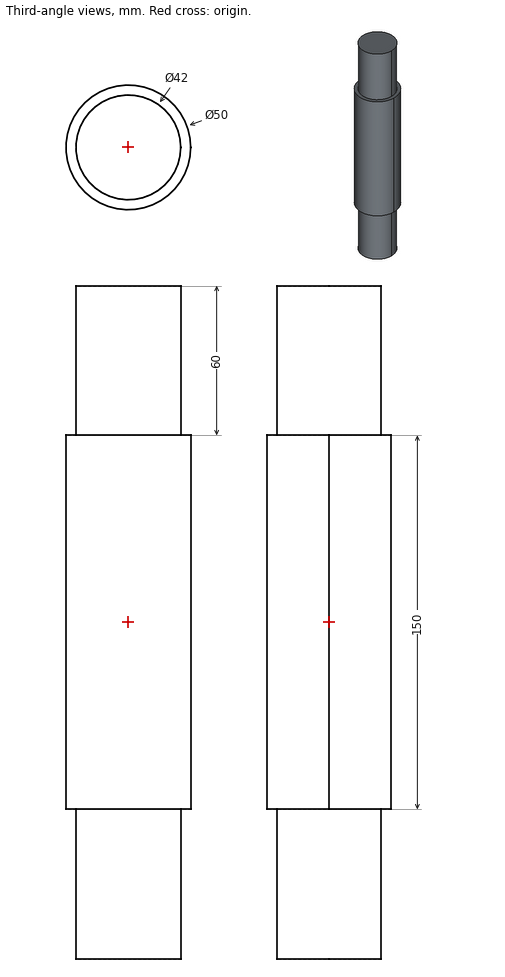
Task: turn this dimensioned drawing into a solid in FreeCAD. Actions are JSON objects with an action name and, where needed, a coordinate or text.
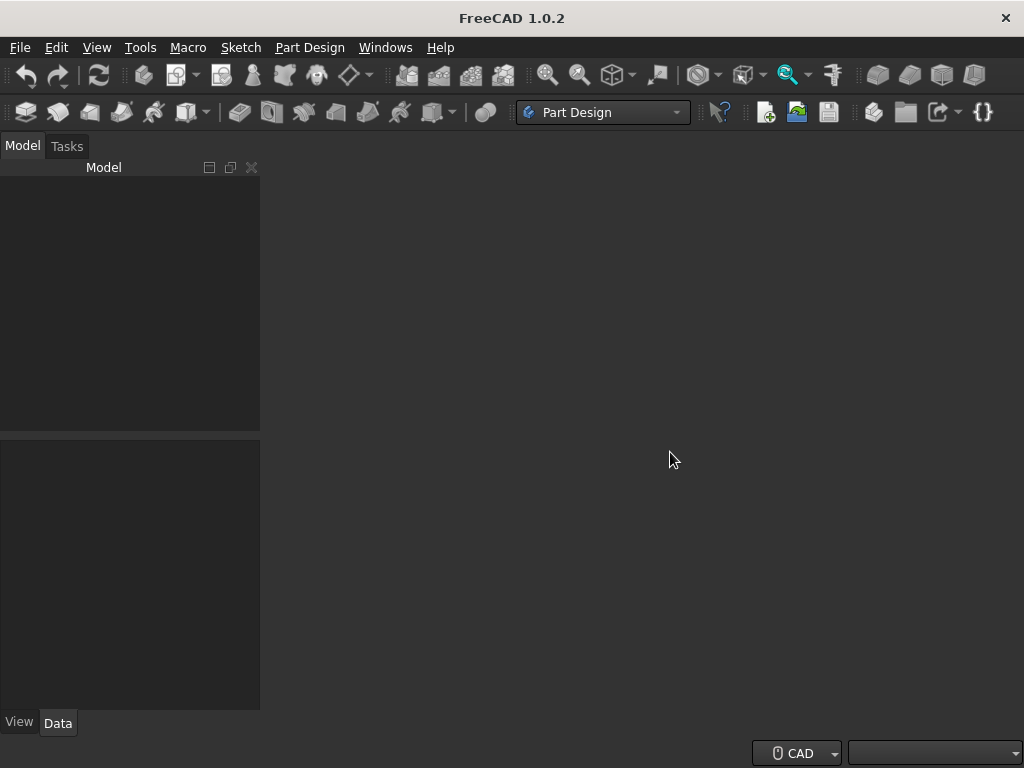
{"action": "left_click", "coordinate": [766, 112]}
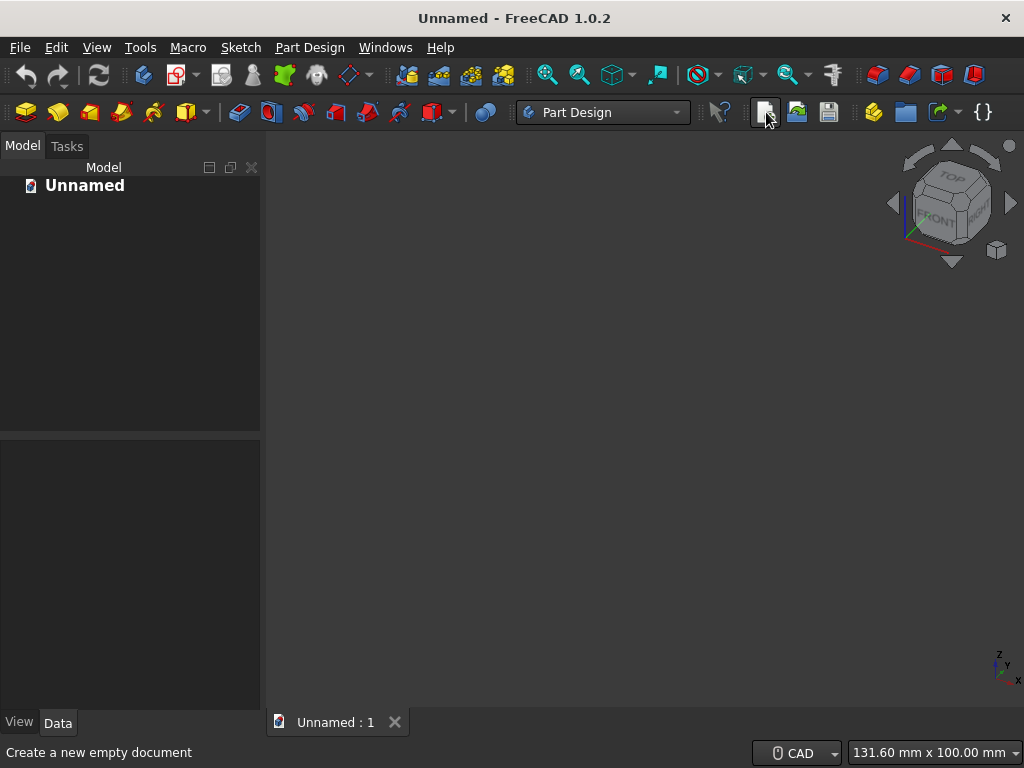
{"action": "left_click", "coordinate": [176, 76]}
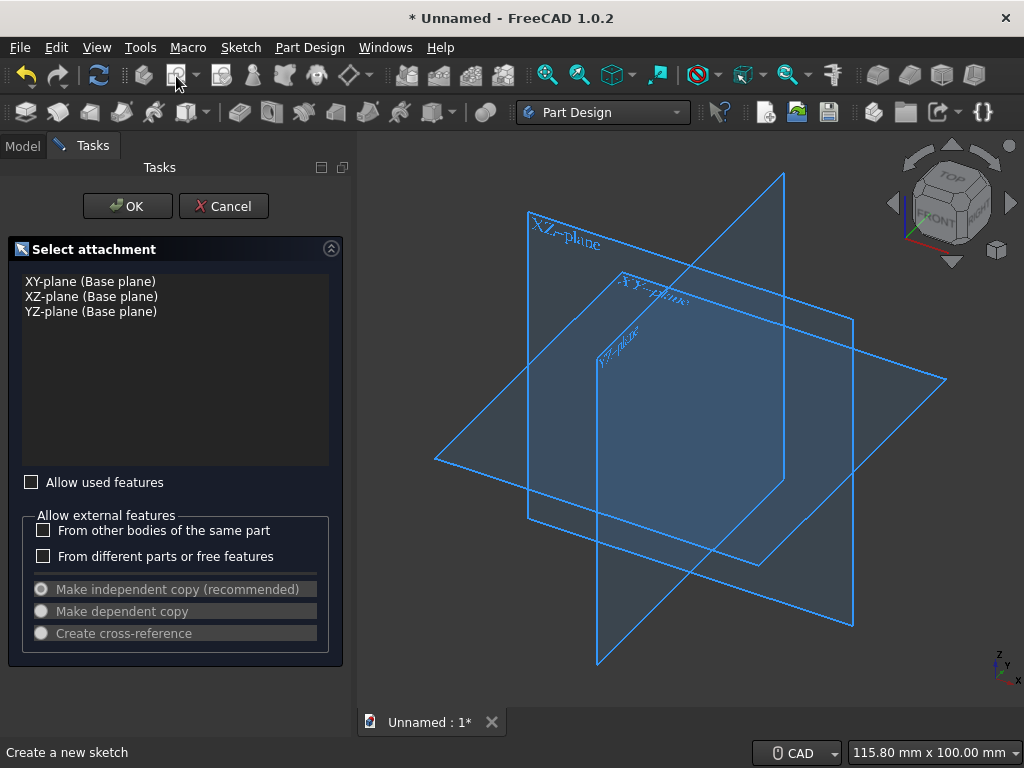
{"action": "left_click", "coordinate": [82, 282]}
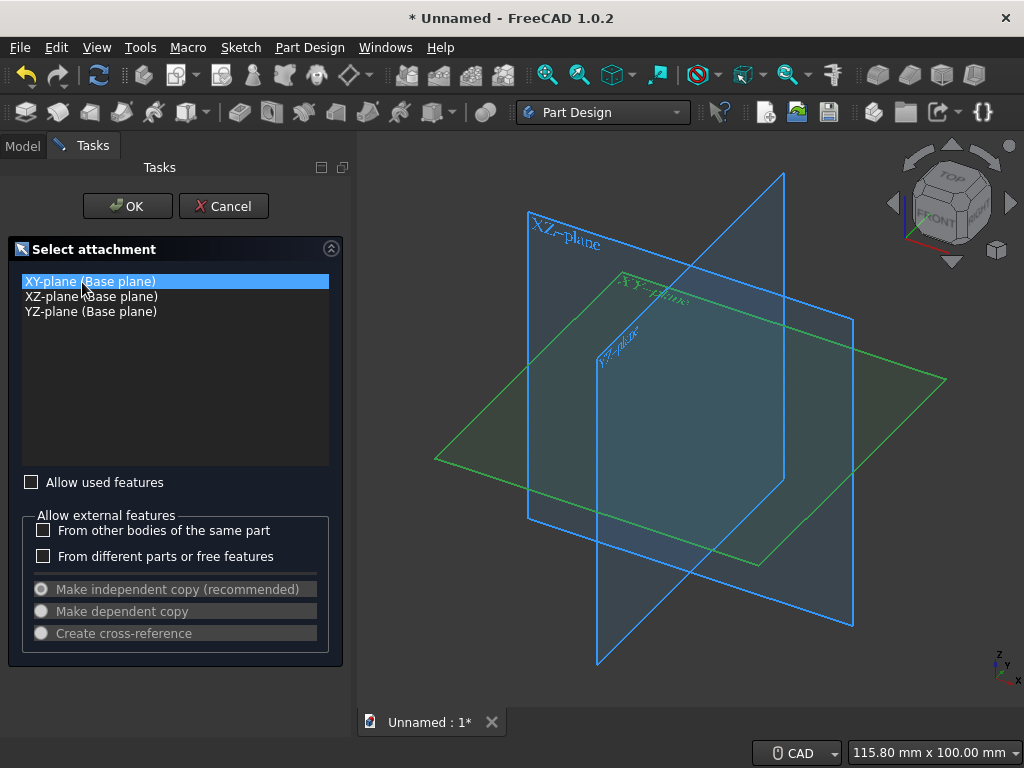
{"action": "left_click", "coordinate": [128, 206]}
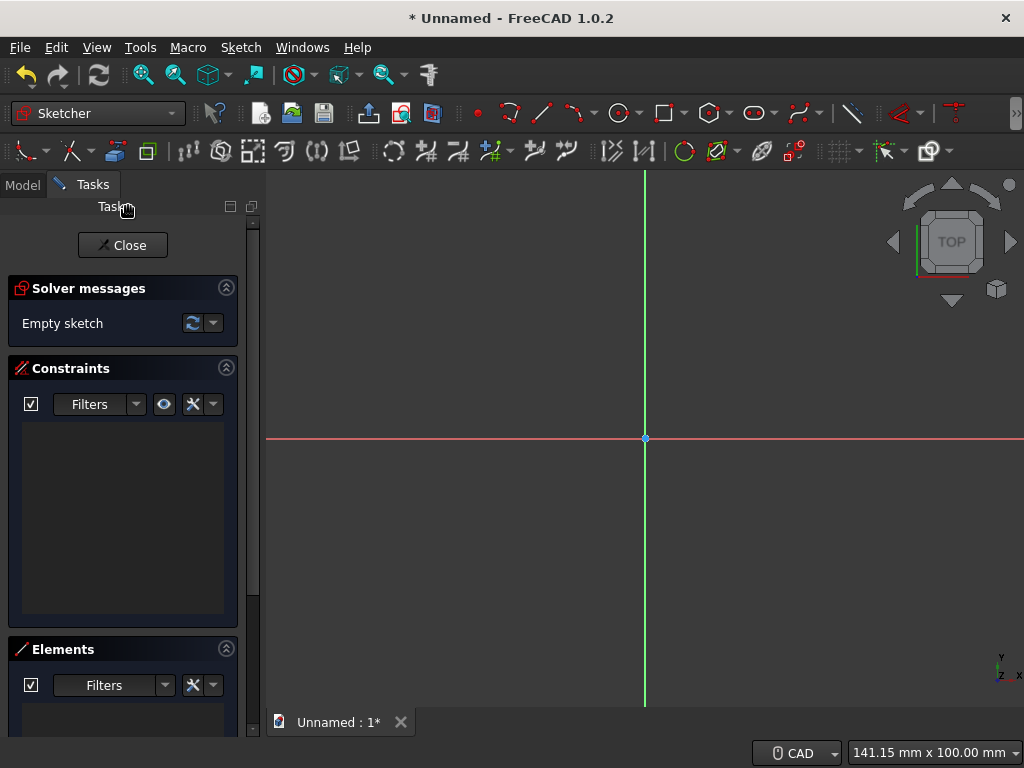
{"action": "left_click", "coordinate": [620, 114]}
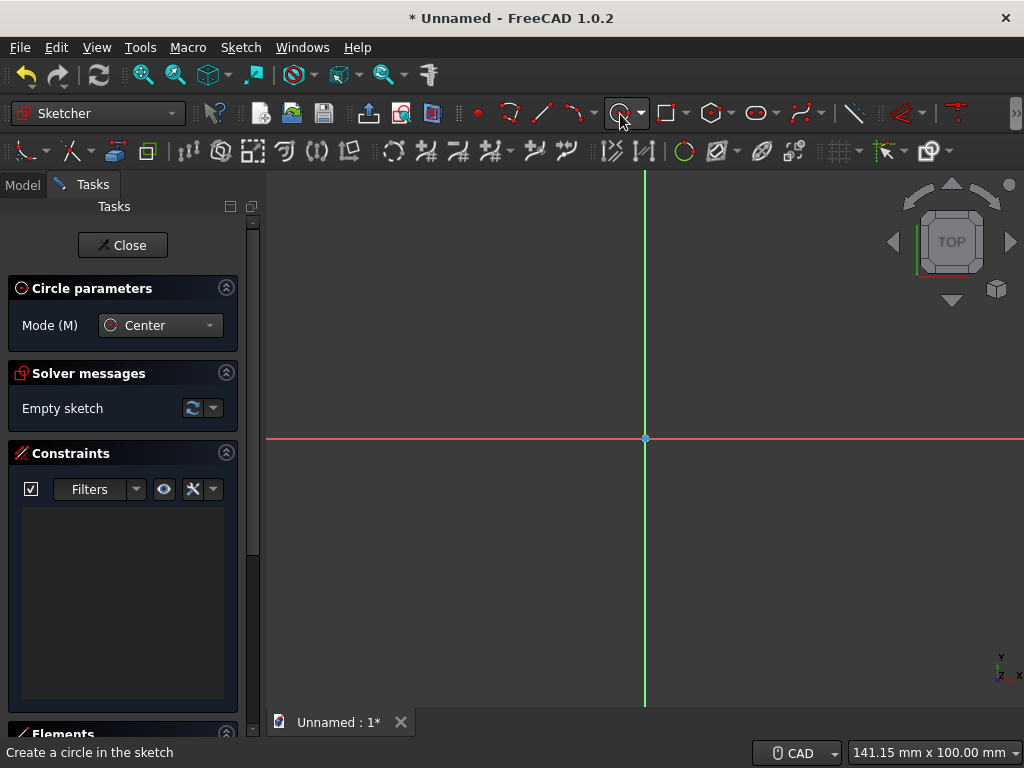
{"action": "left_click", "coordinate": [645, 438]}
{"action": "left_click", "coordinate": [740, 344]}
{"action": "key", "text": "Escape"}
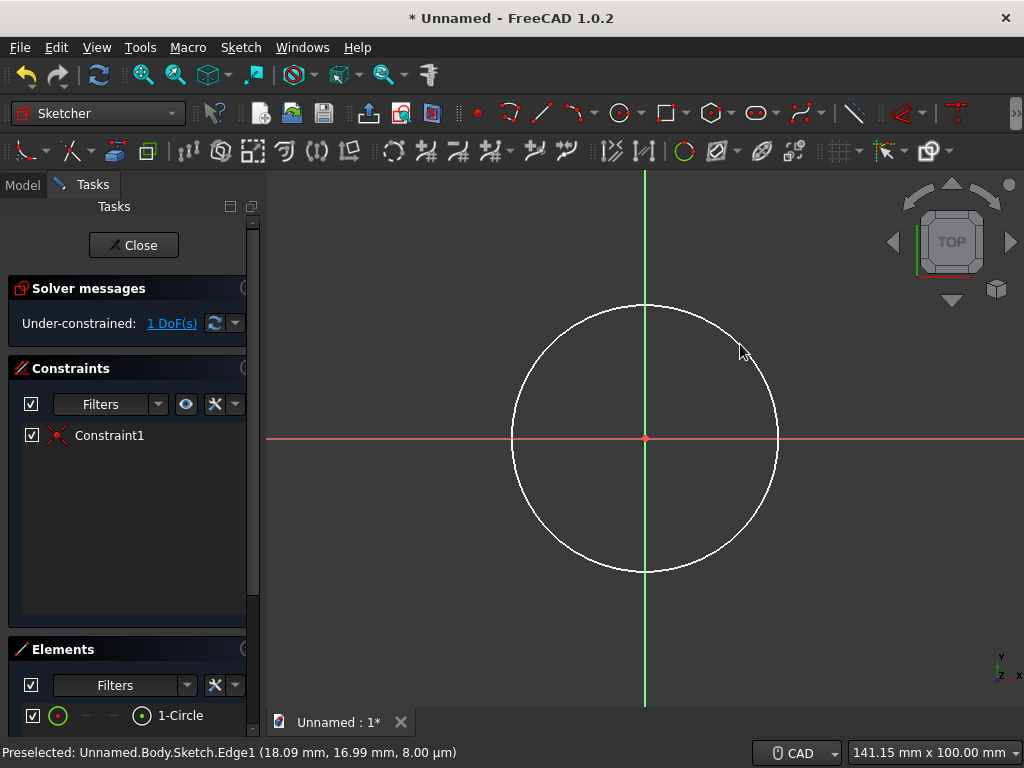
{"action": "left_click", "coordinate": [739, 344]}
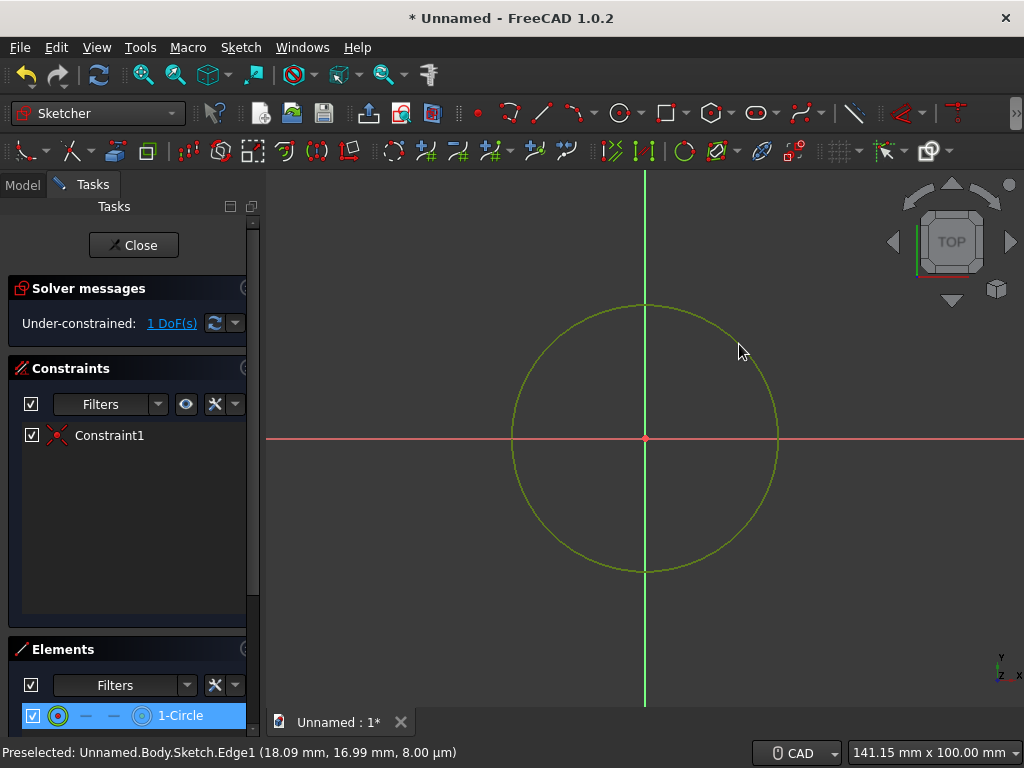
{"action": "key", "text": "k o"}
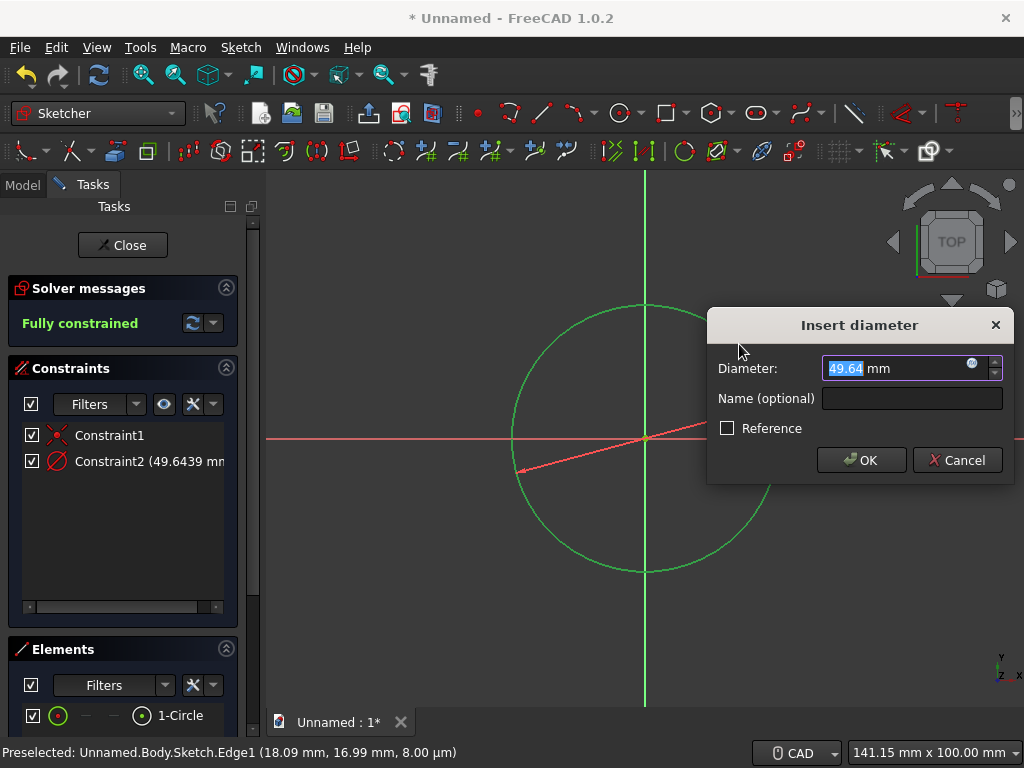
{"action": "type", "text": "50"}
{"action": "key", "text": "Return"}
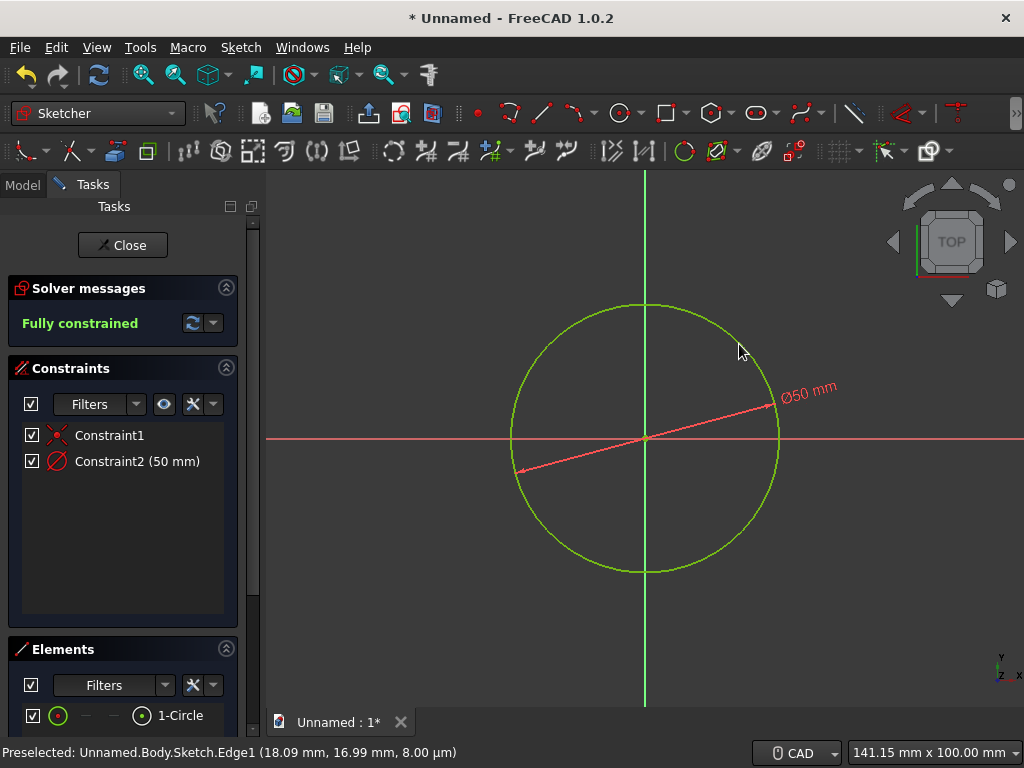
{"action": "left_click", "coordinate": [123, 245]}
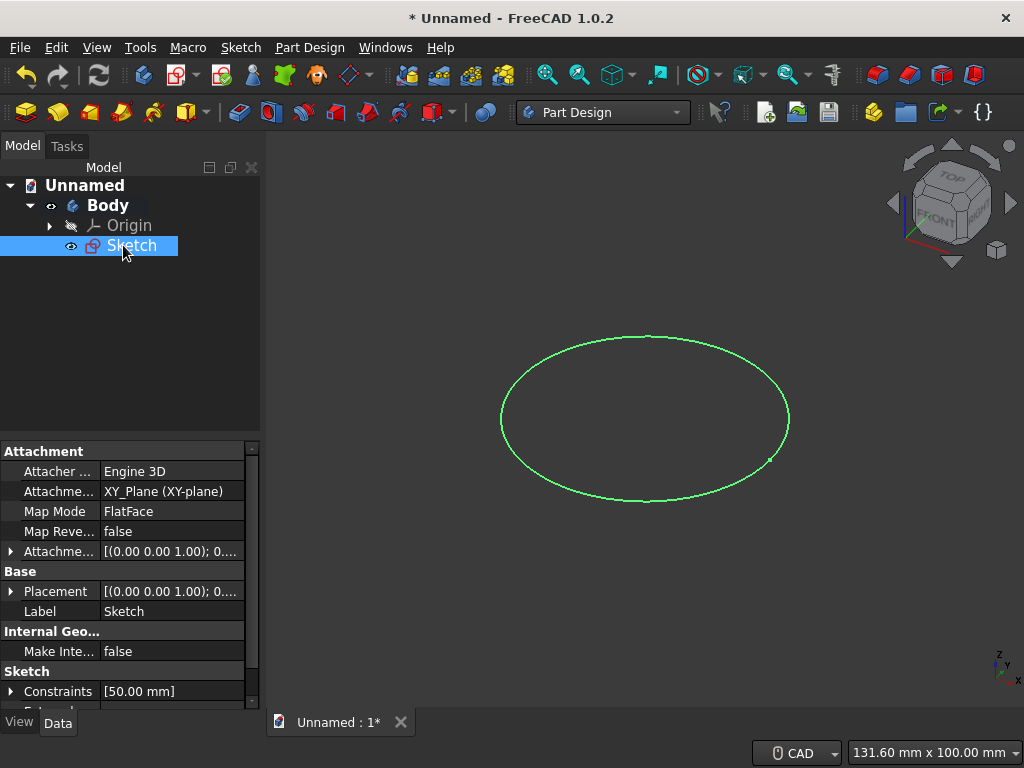
{"action": "left_click", "coordinate": [26, 112]}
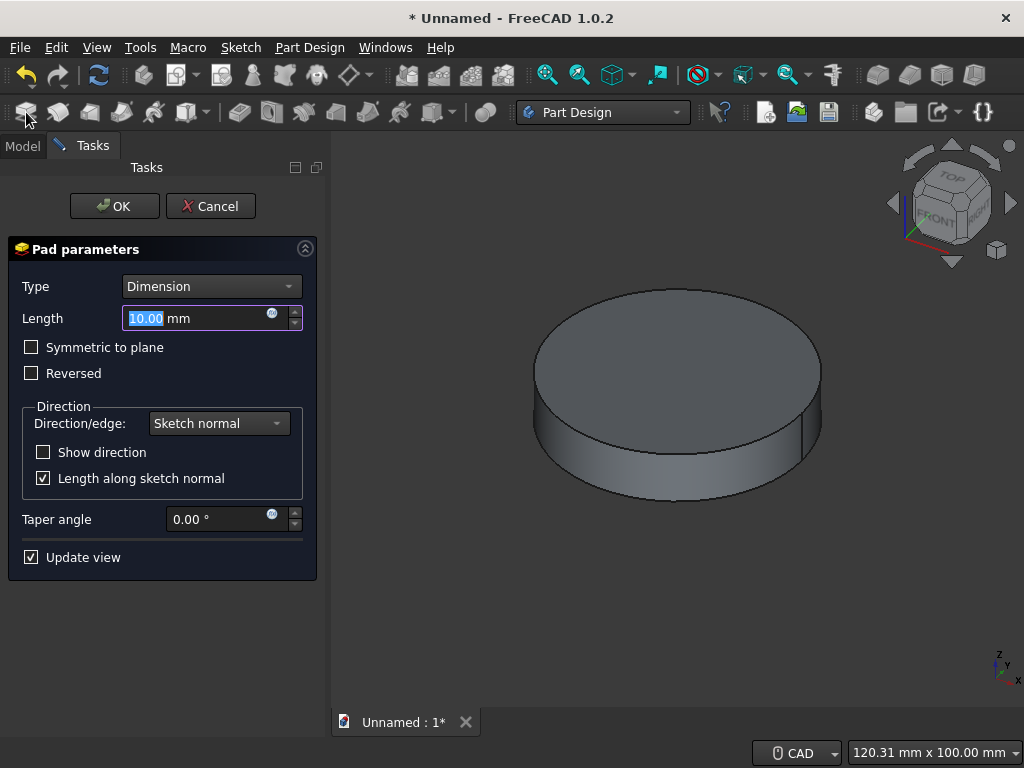
{"action": "type", "text": "150"}
{"action": "key", "text": "Tab"}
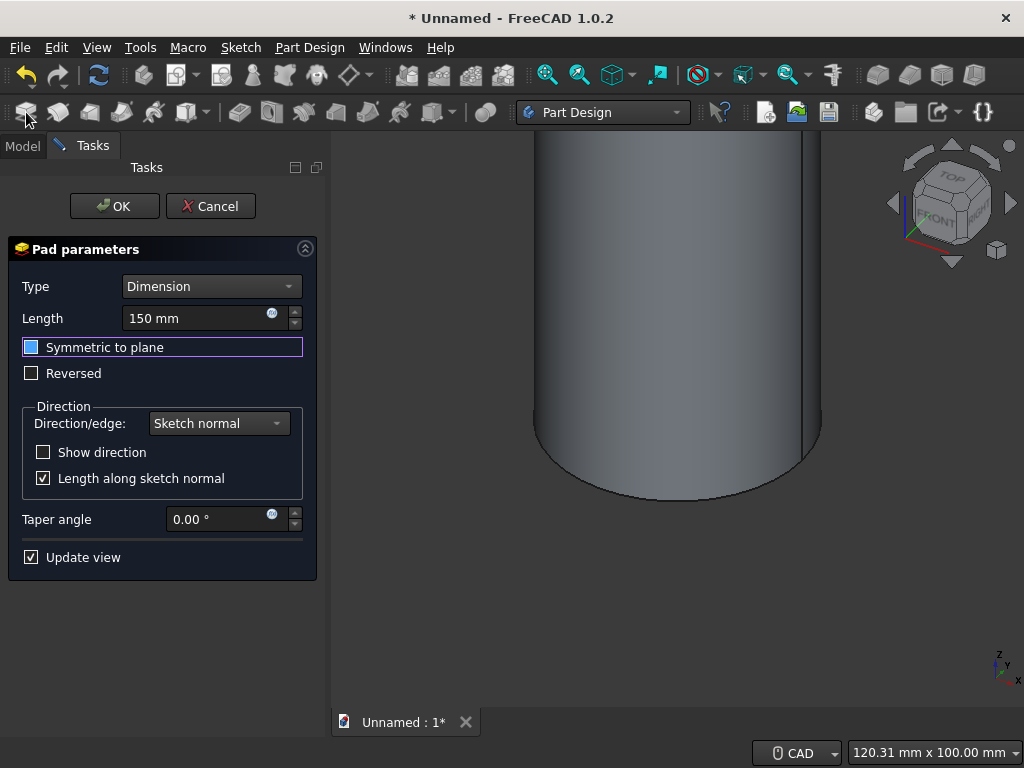
{"action": "left_click", "coordinate": [30, 347]}